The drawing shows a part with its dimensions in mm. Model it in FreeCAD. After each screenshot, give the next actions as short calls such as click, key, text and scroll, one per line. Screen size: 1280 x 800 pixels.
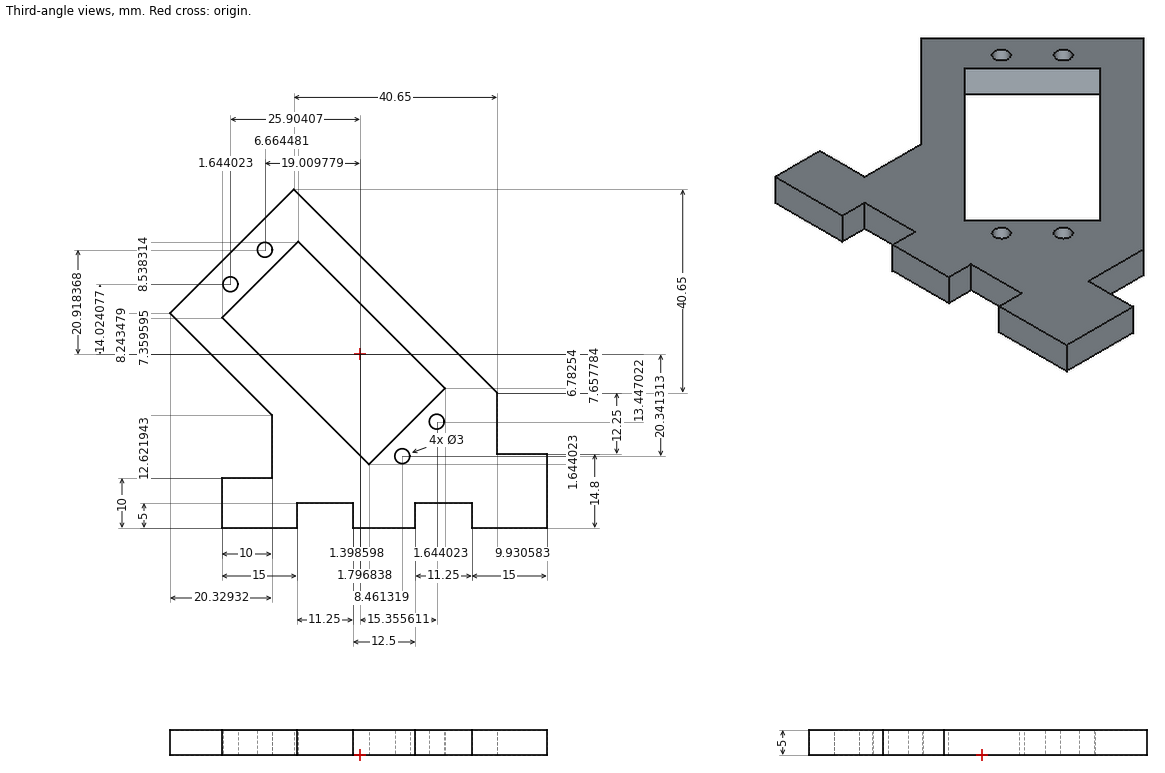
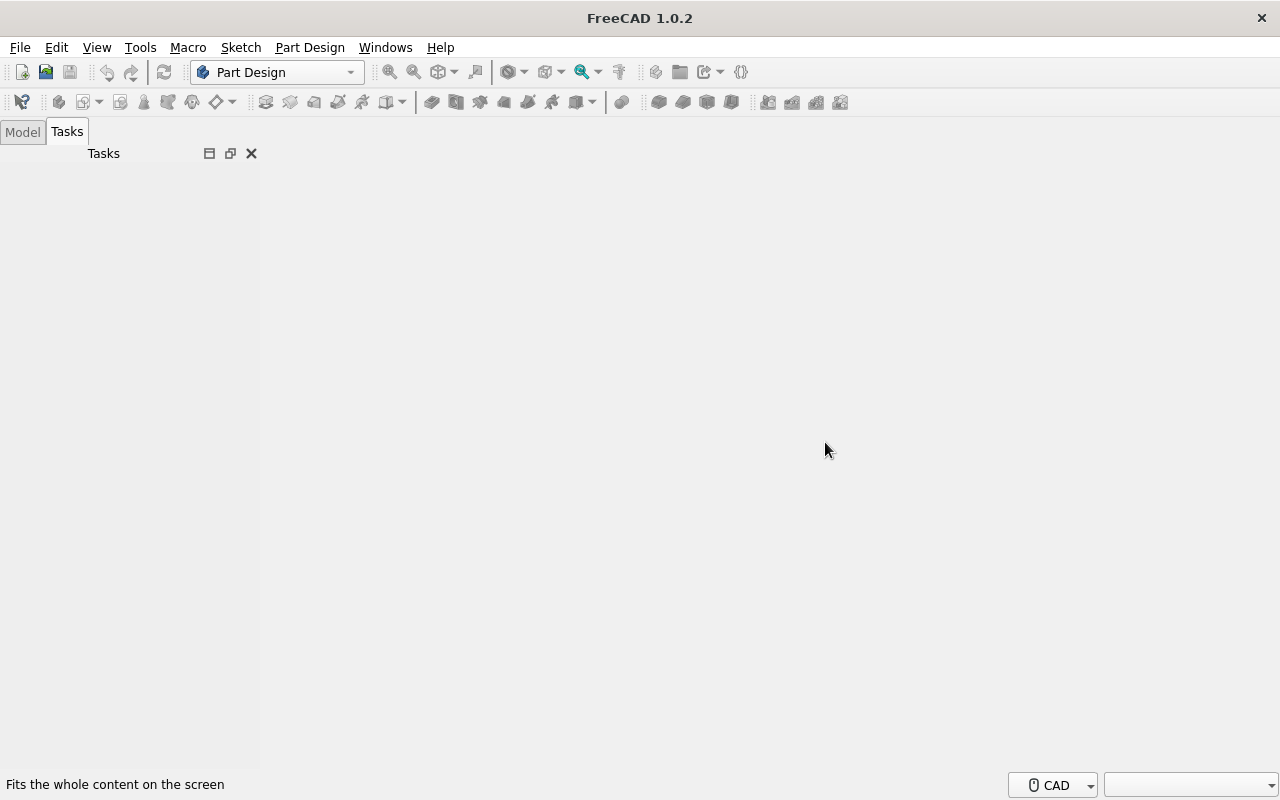
click(22, 72)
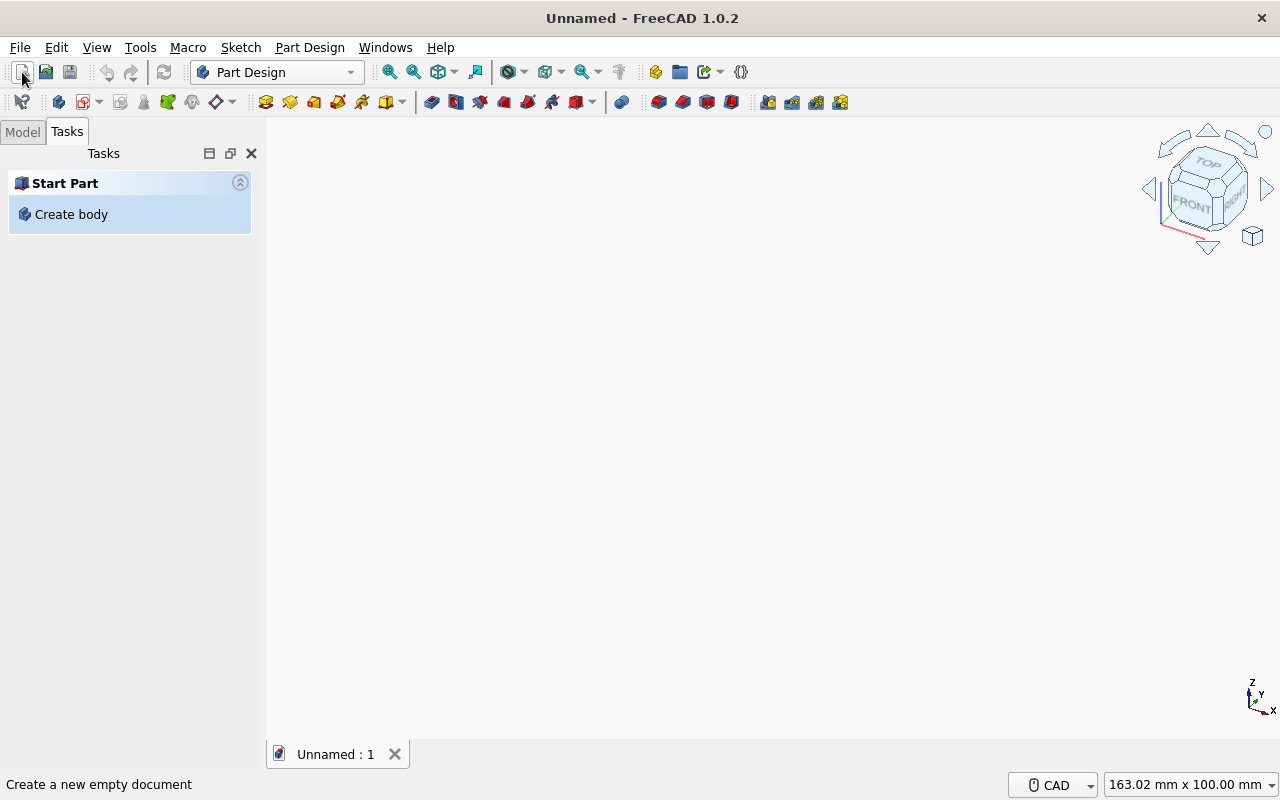
click(84, 102)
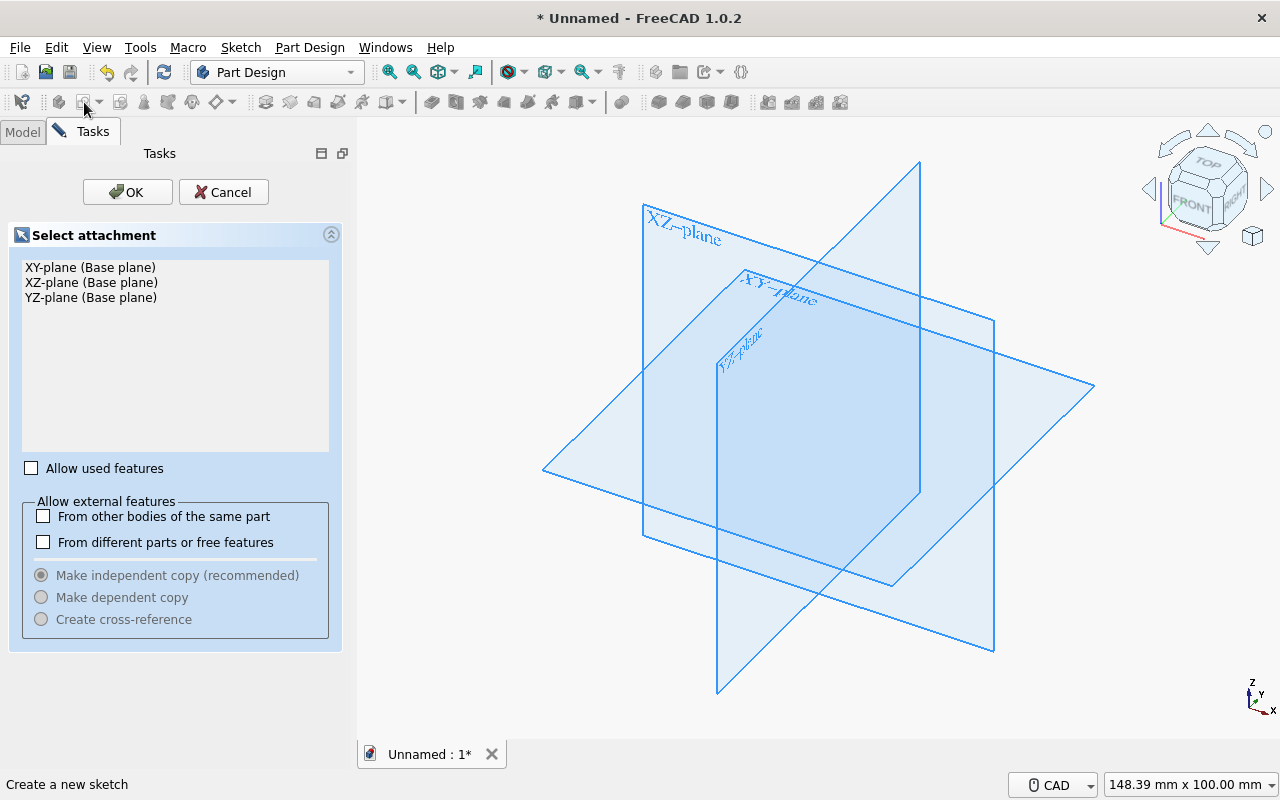
click(82, 268)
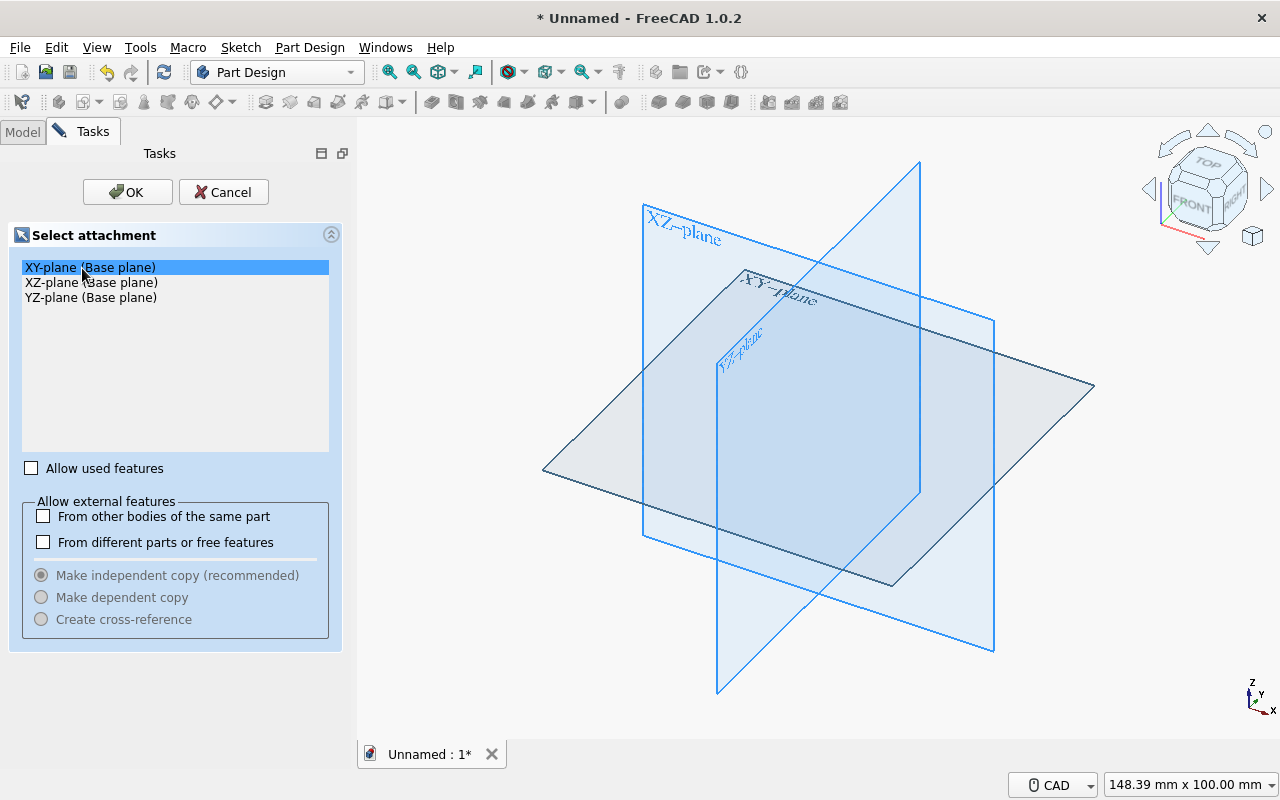
click(128, 192)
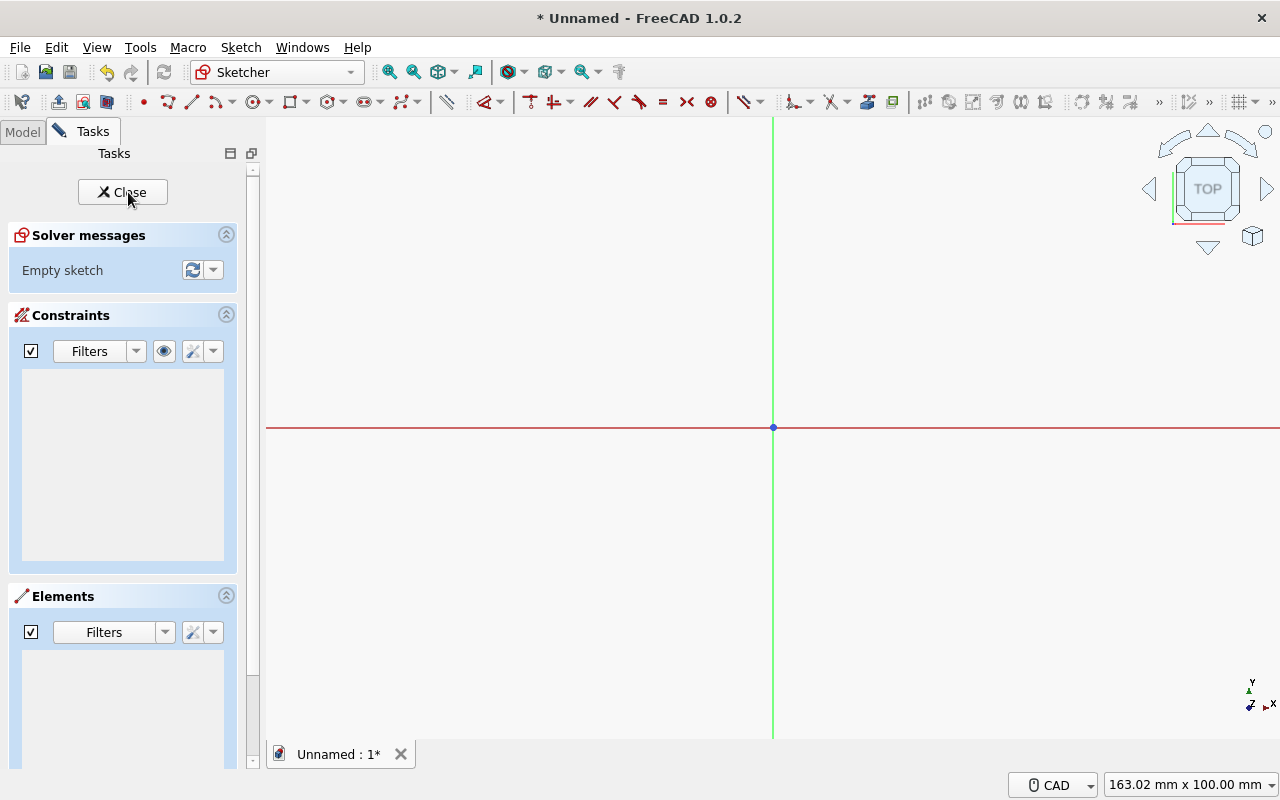
key(g)
key(m)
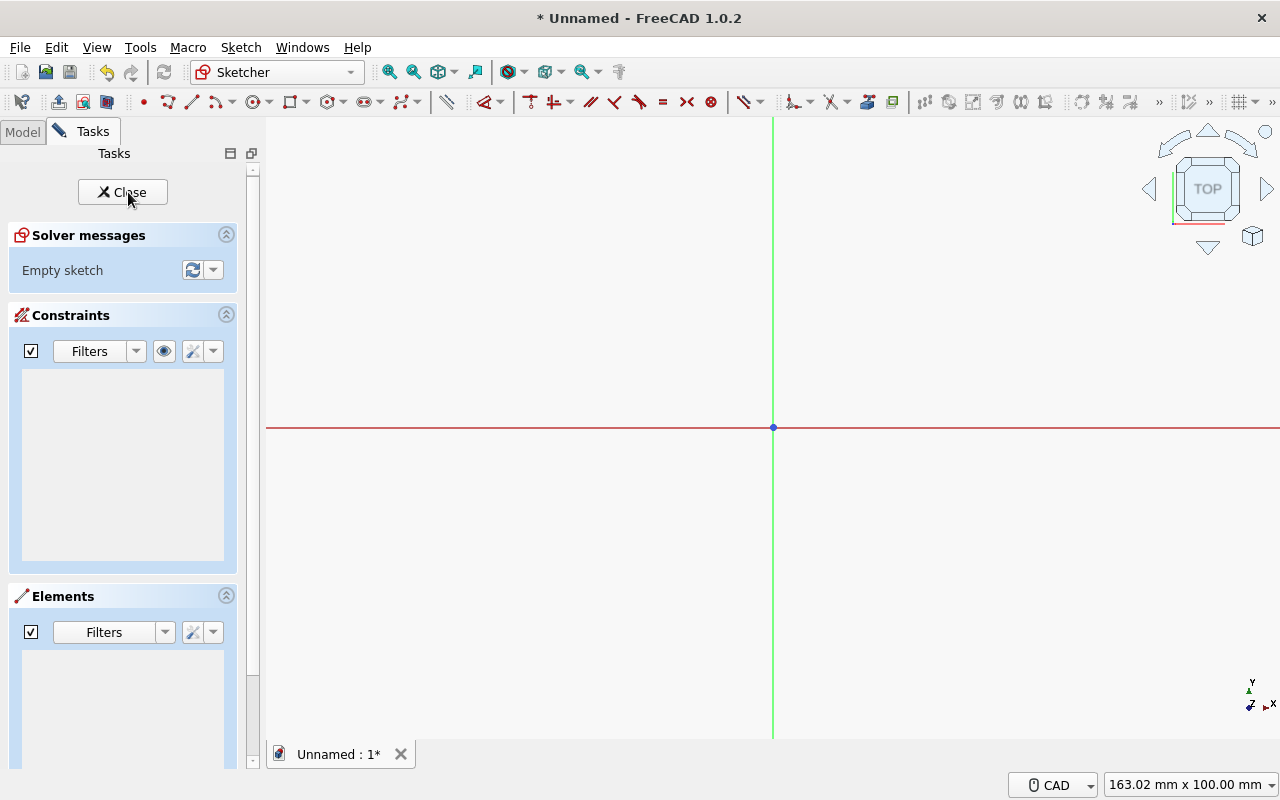
click(663, 503)
click(663, 582)
click(601, 582)
click(601, 644)
click(694, 644)
click(694, 613)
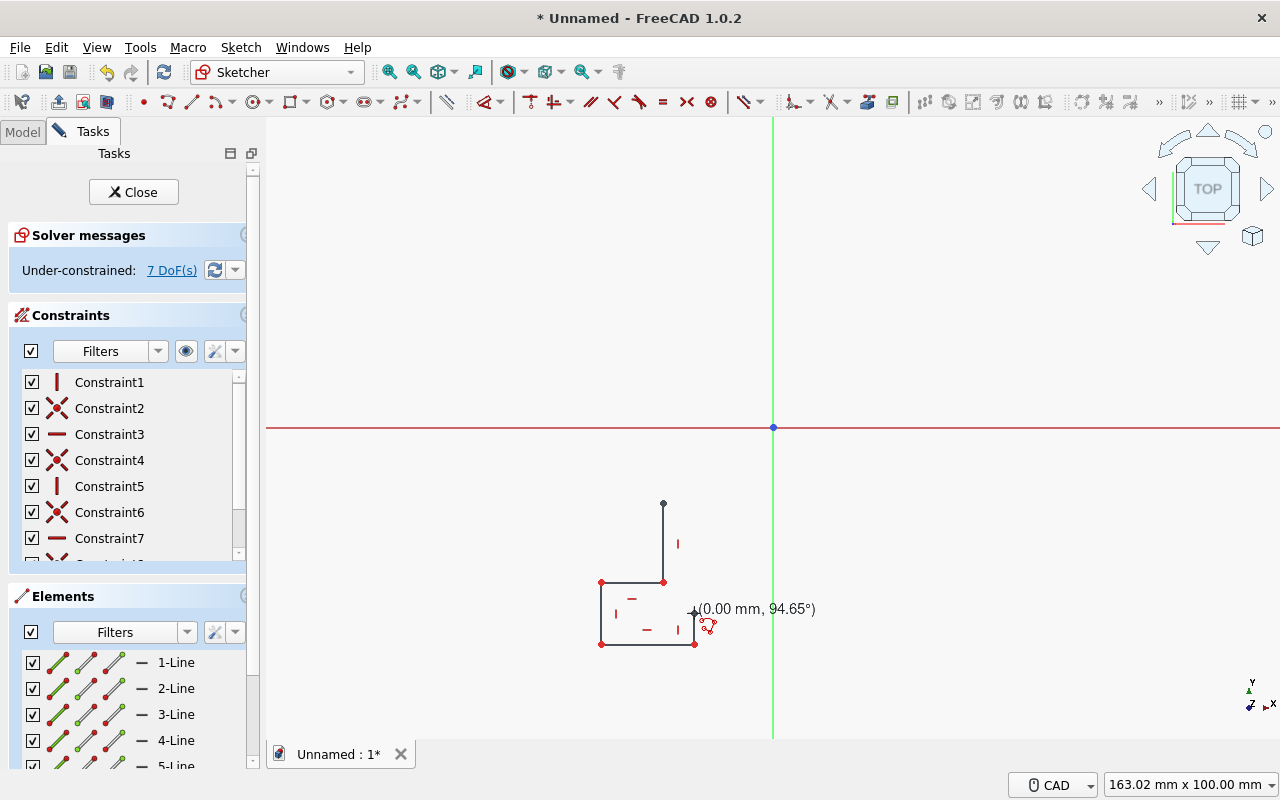
scroll(764, 613, up, 4)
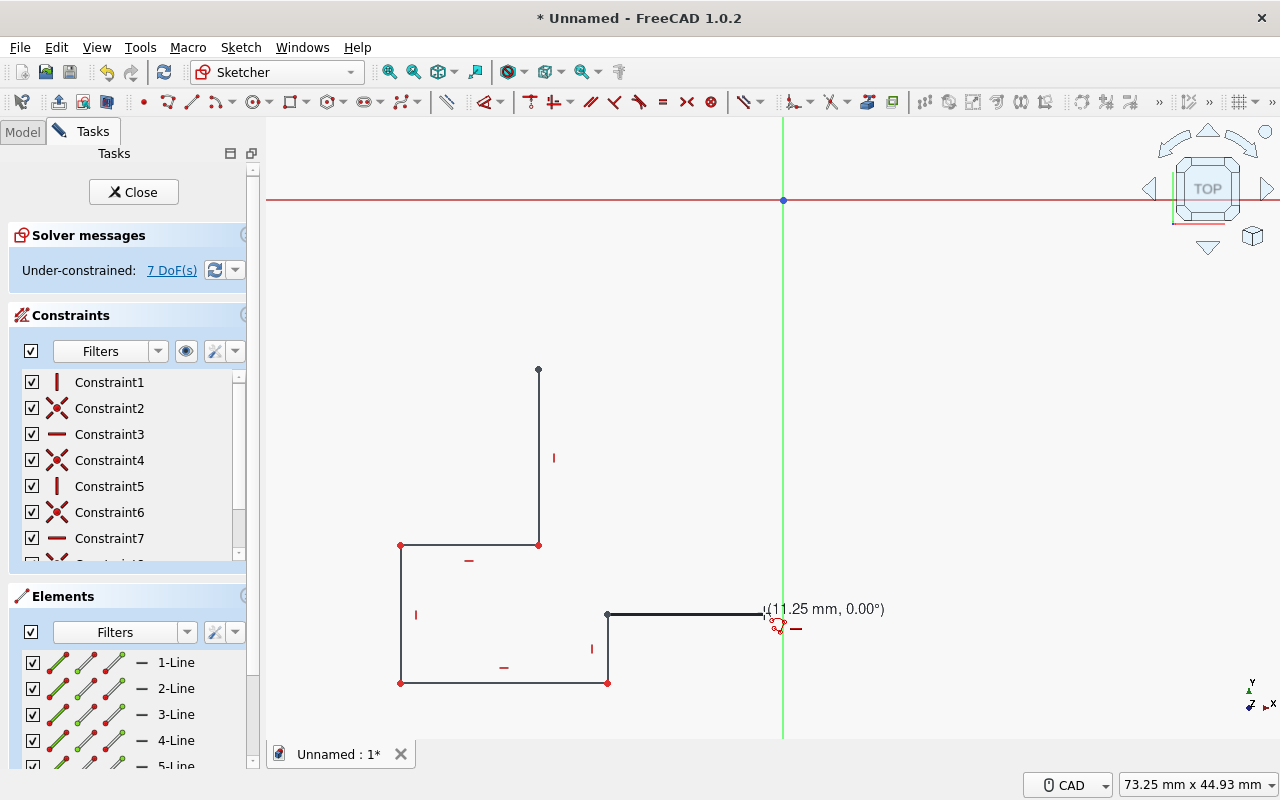
click(764, 612)
click(764, 681)
click(937, 681)
click(937, 612)
click(1093, 612)
click(1093, 681)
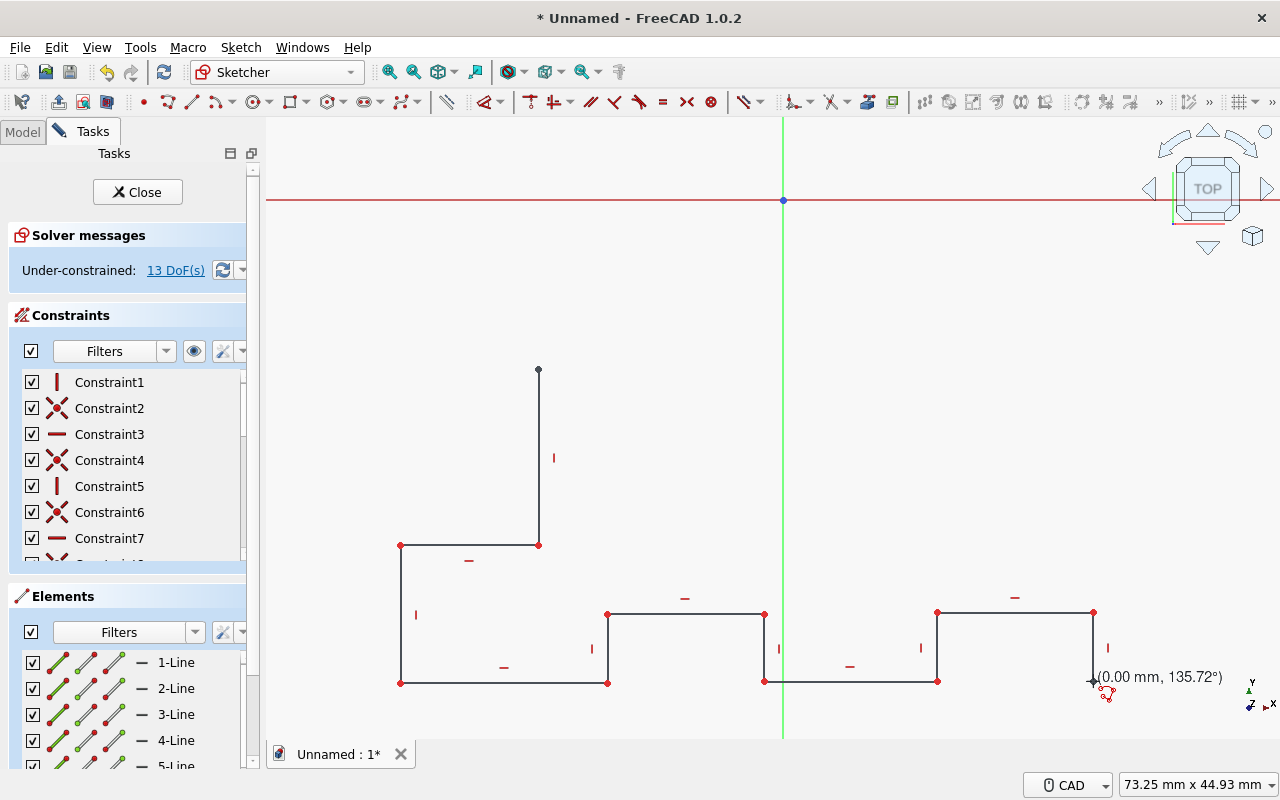
scroll(644, 604, down, 4)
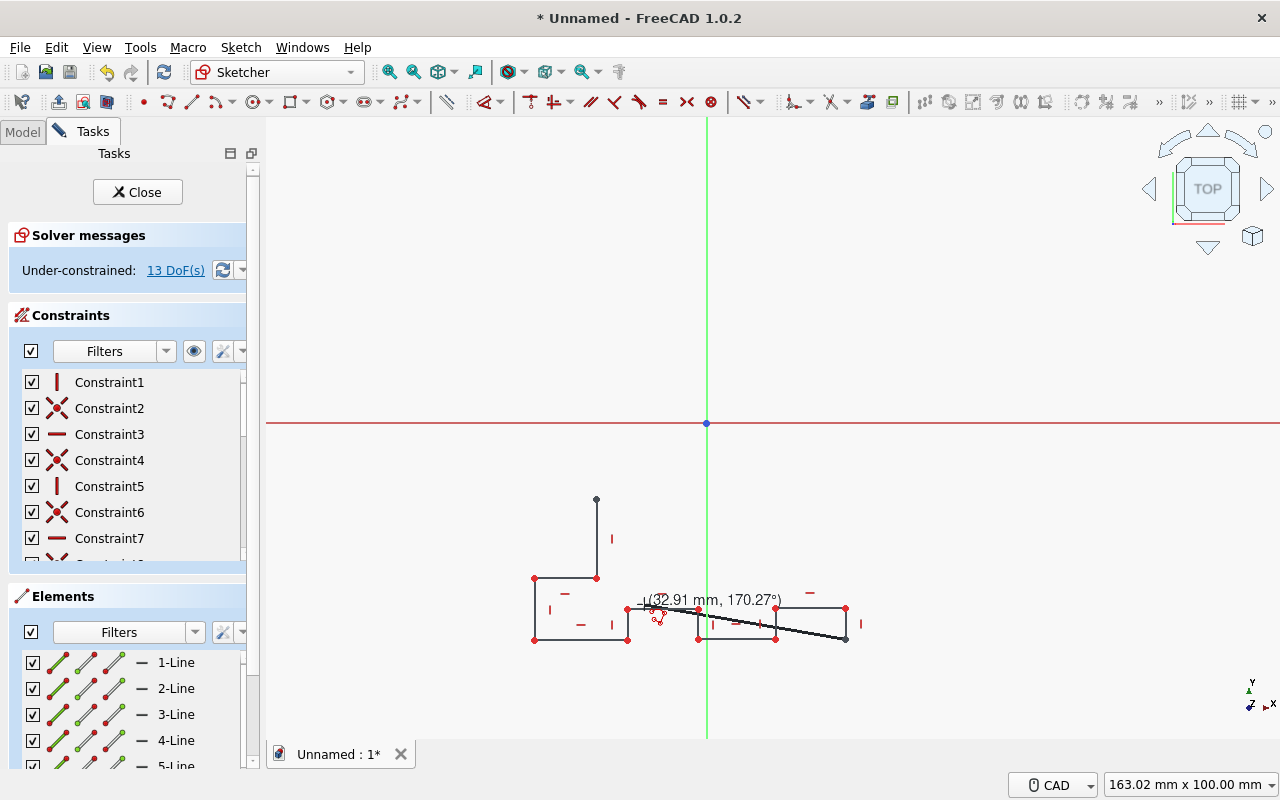
click(939, 639)
click(939, 547)
click(877, 547)
click(877, 471)
click(625, 218)
click(471, 372)
click(597, 499)